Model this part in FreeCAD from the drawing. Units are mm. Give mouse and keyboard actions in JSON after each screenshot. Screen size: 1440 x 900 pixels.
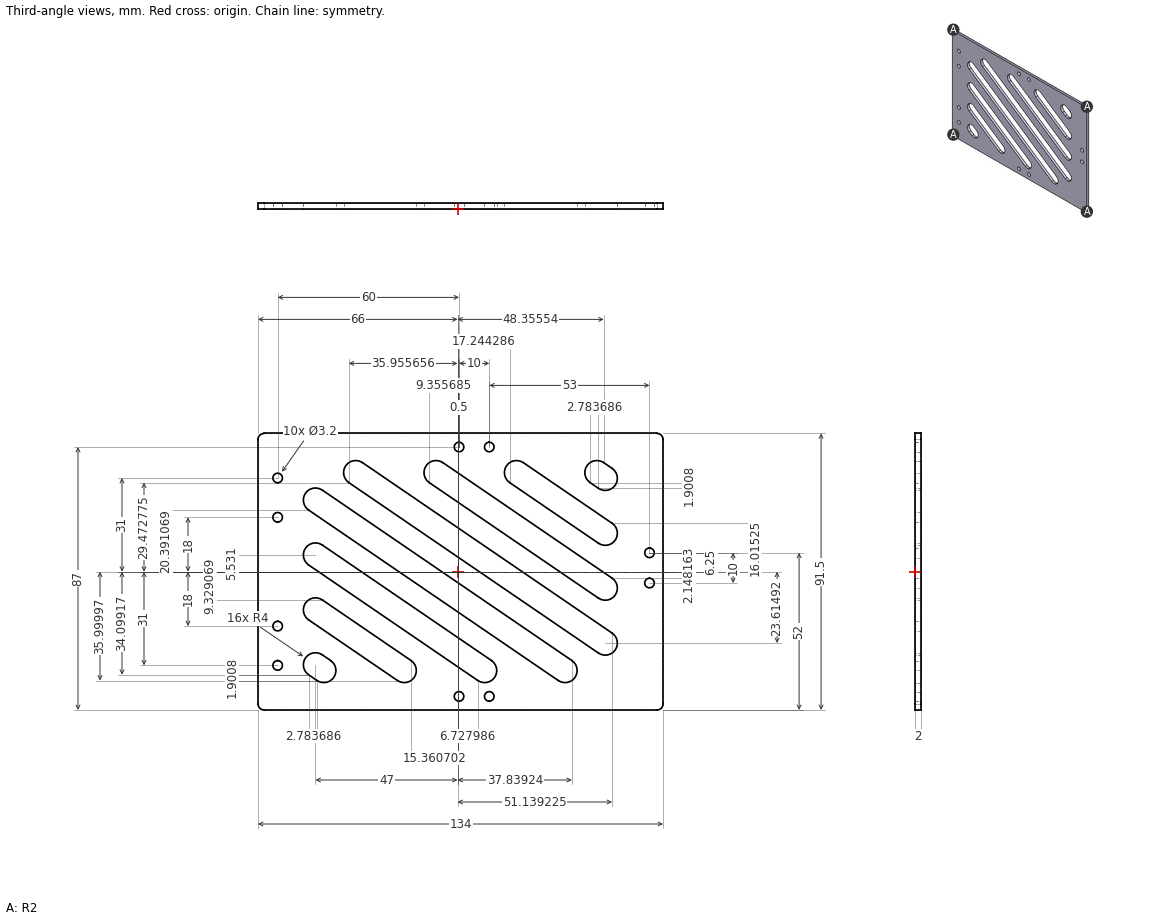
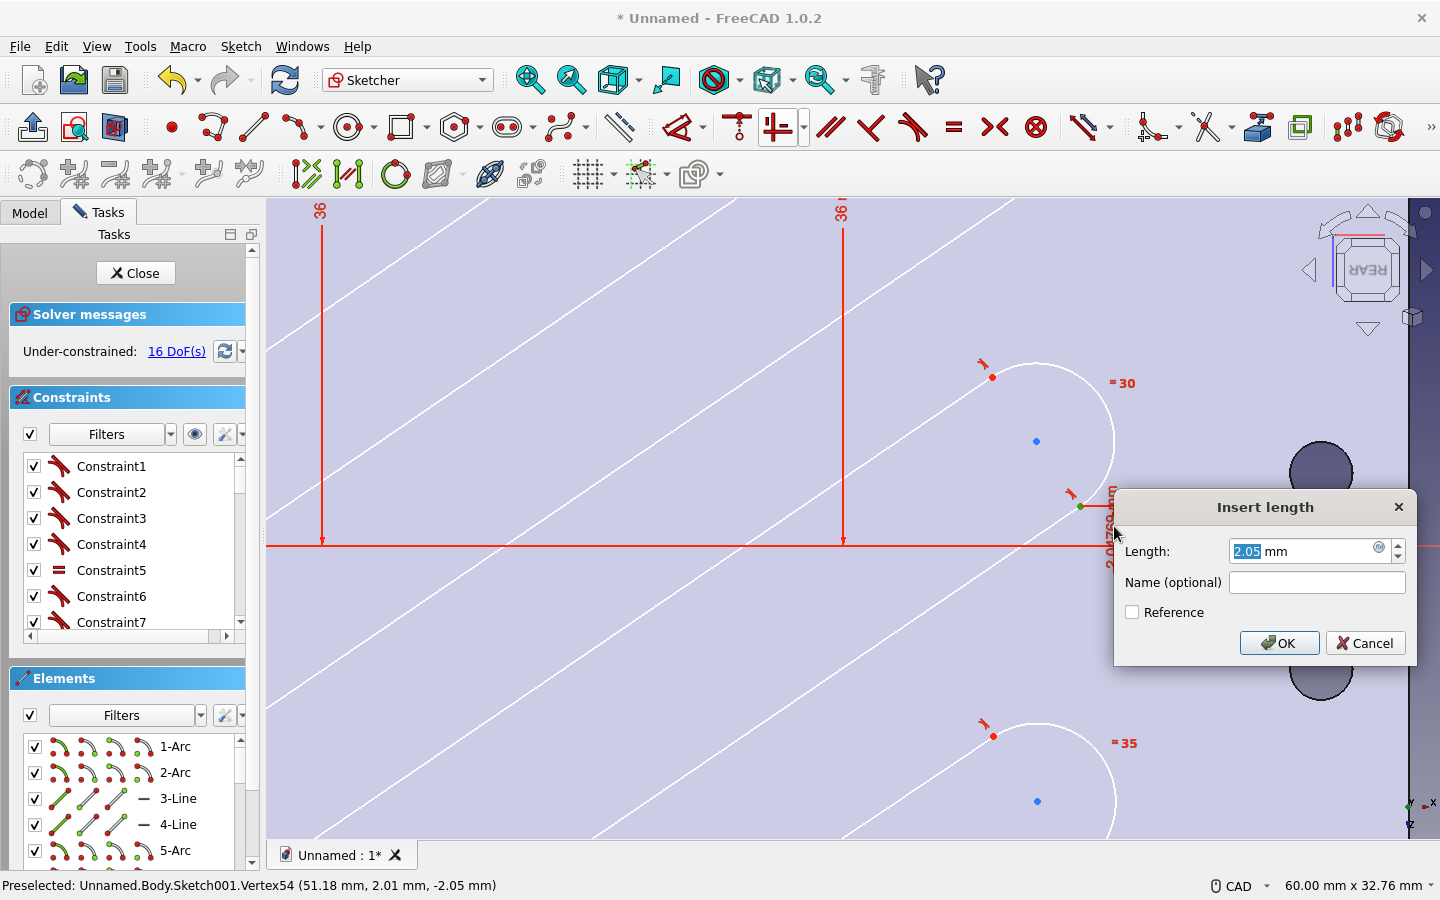
{"action": "type", "text": "2.148163"}
{"action": "key", "text": "Return"}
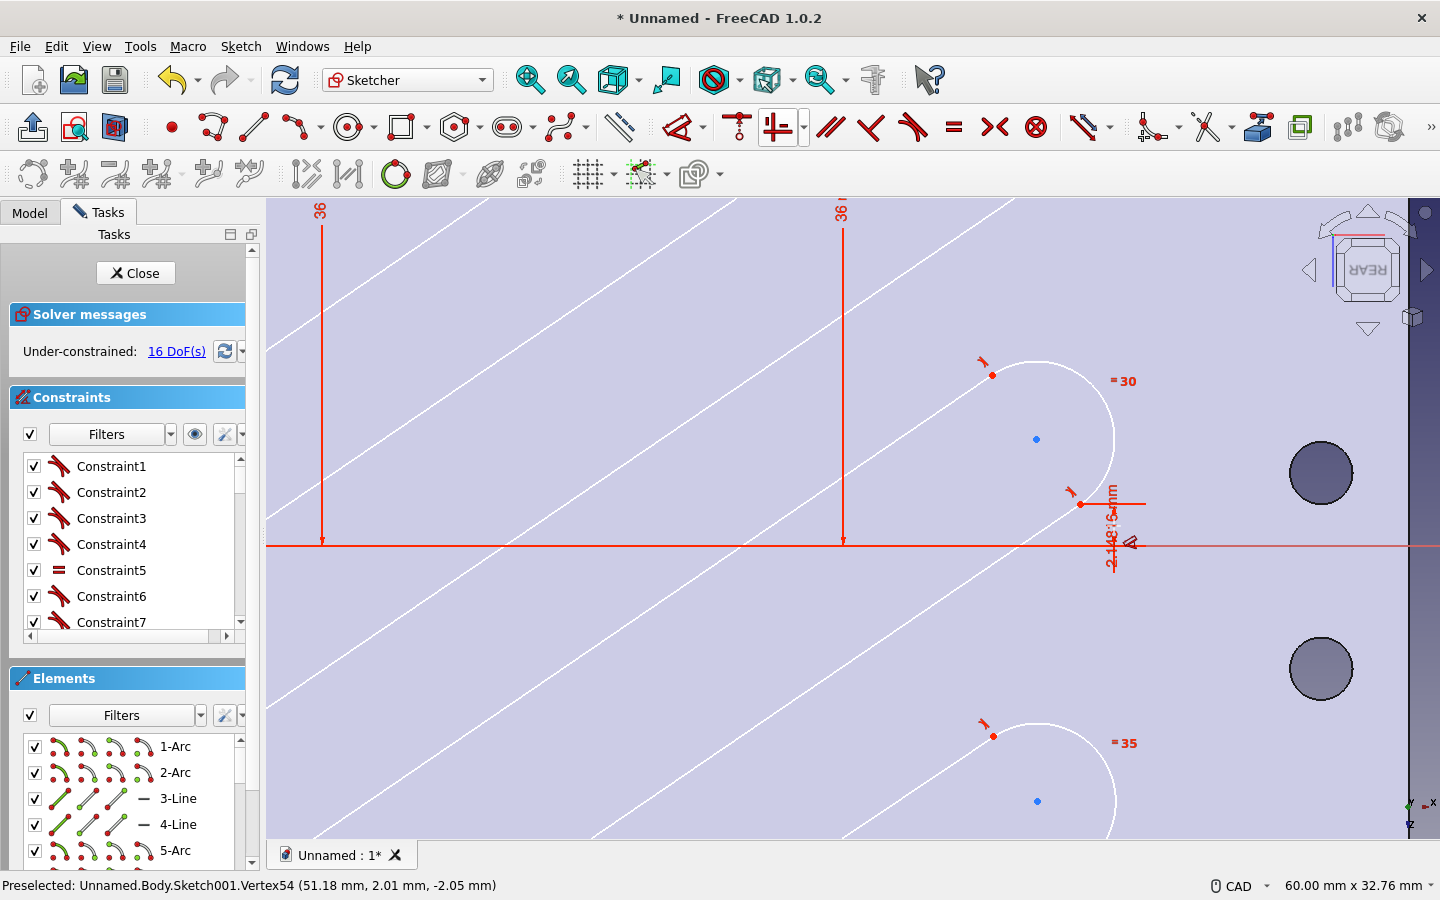
{"action": "scroll", "coordinate": [1081, 506], "scroll_direction": "down", "scroll_amount": 6}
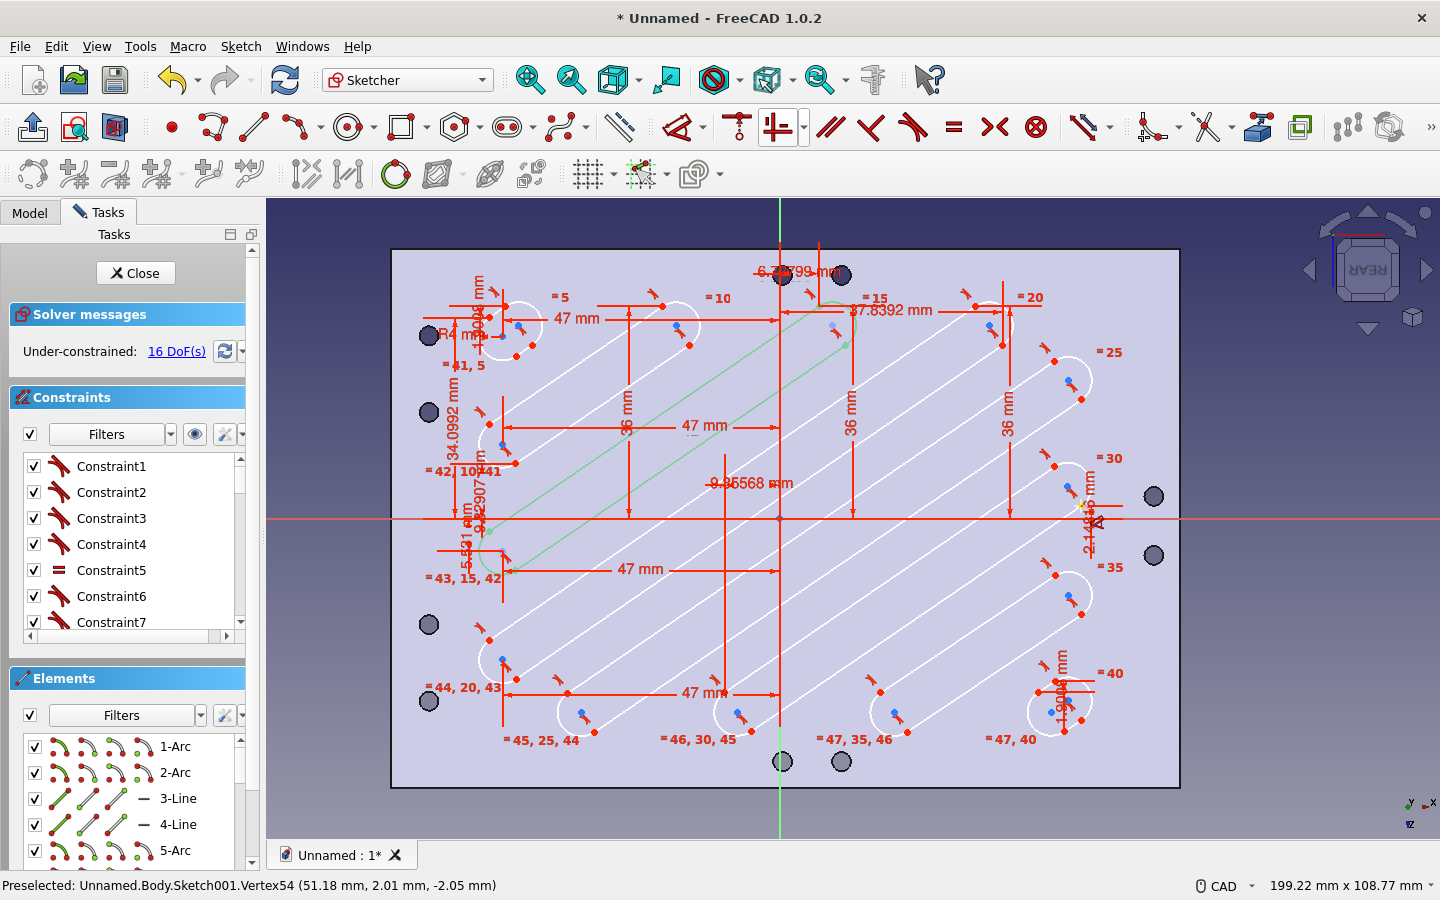
{"action": "left_click", "coordinate": [1082, 615]}
{"action": "left_click", "coordinate": [1116, 567]}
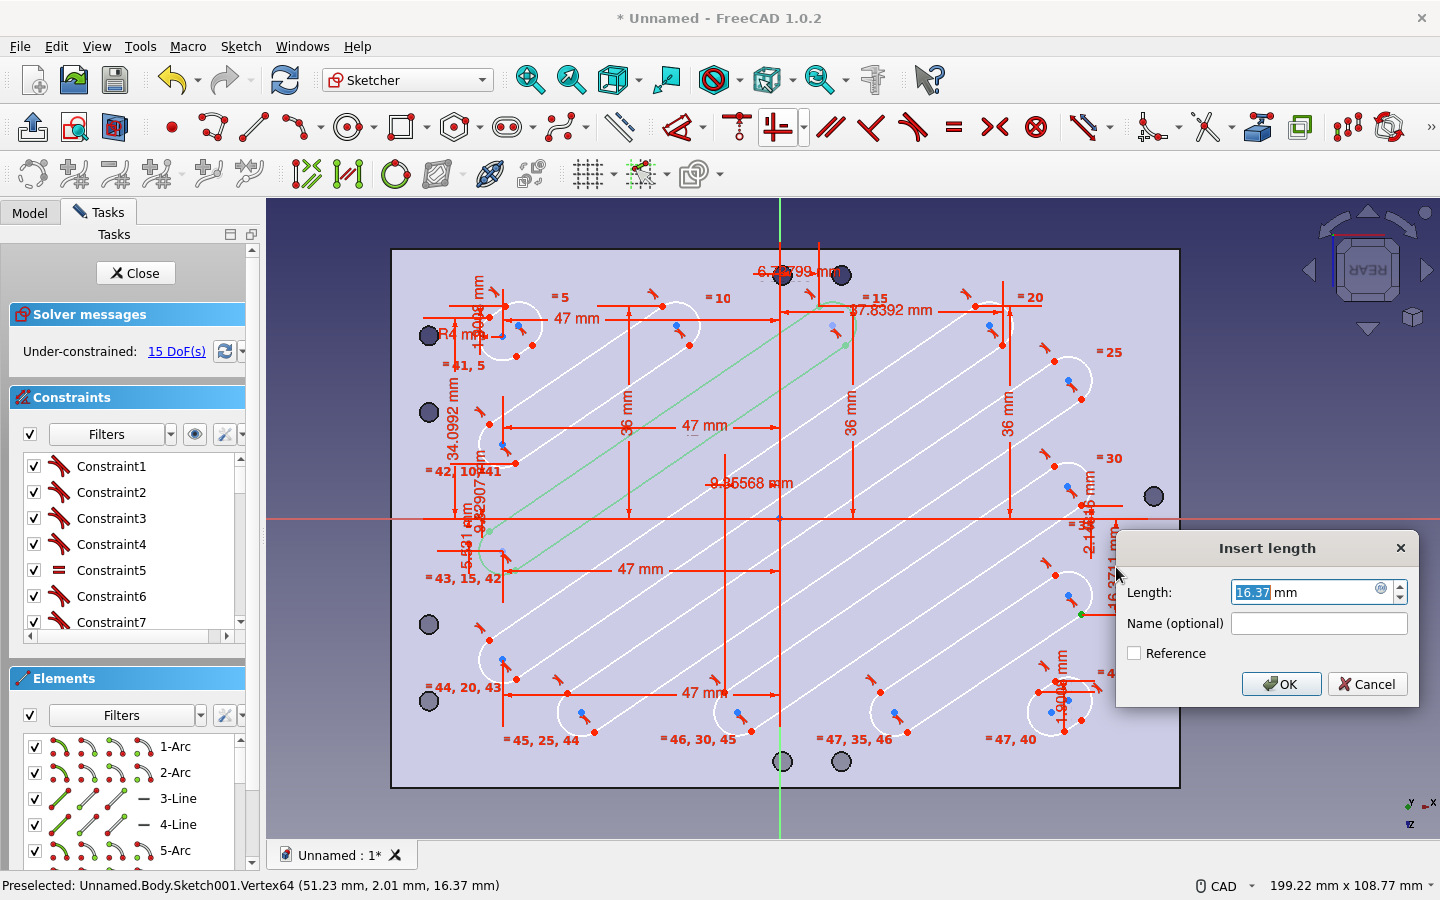
{"action": "type", "text": "16.01525"}
{"action": "key", "text": "Return"}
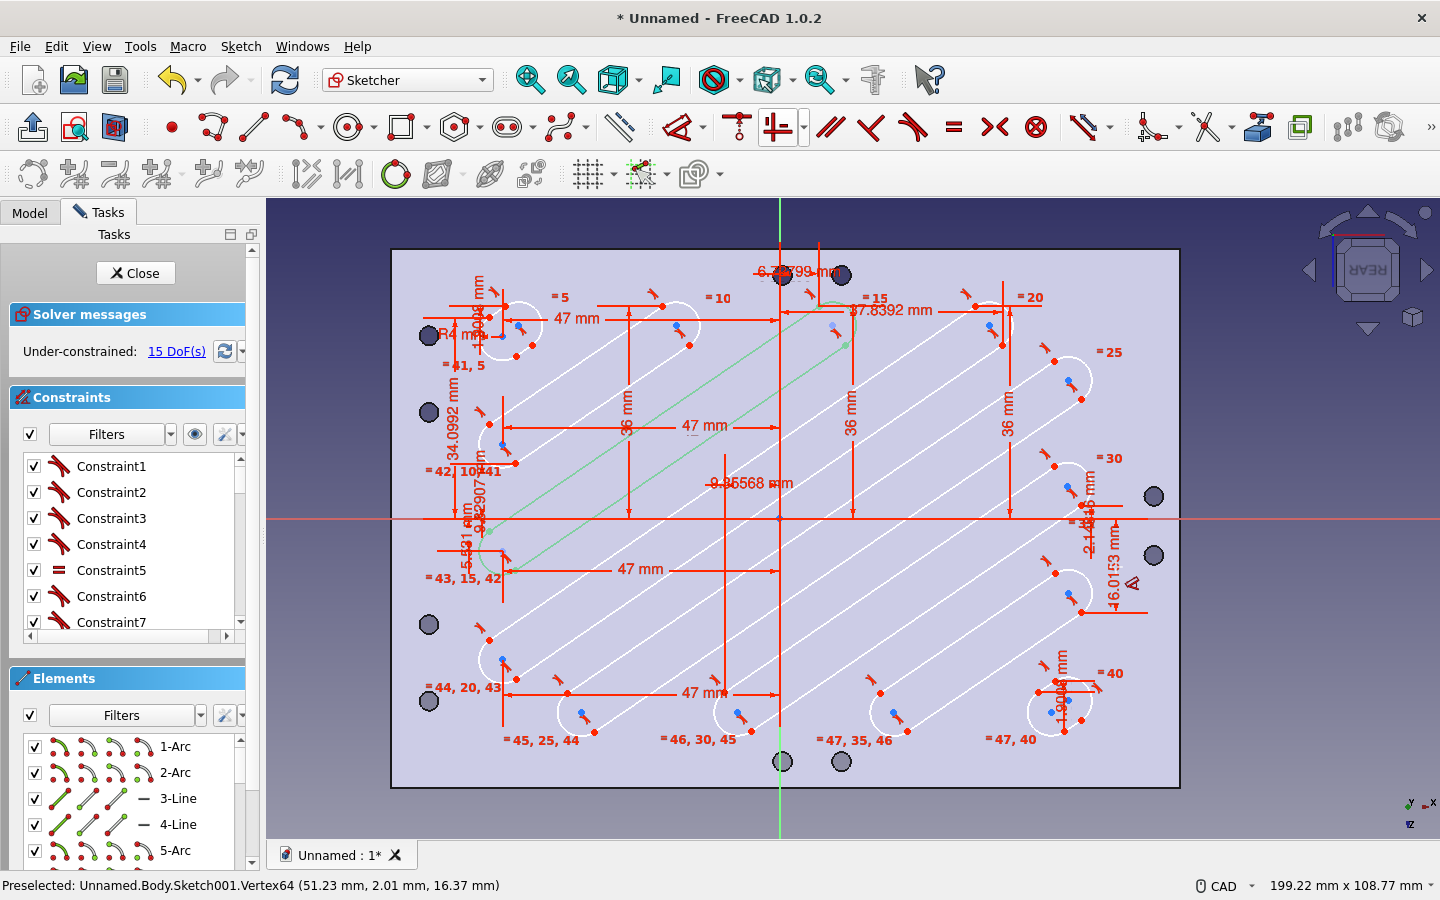
{"action": "left_click", "coordinate": [1064, 732]}
{"action": "left_click", "coordinate": [922, 766]}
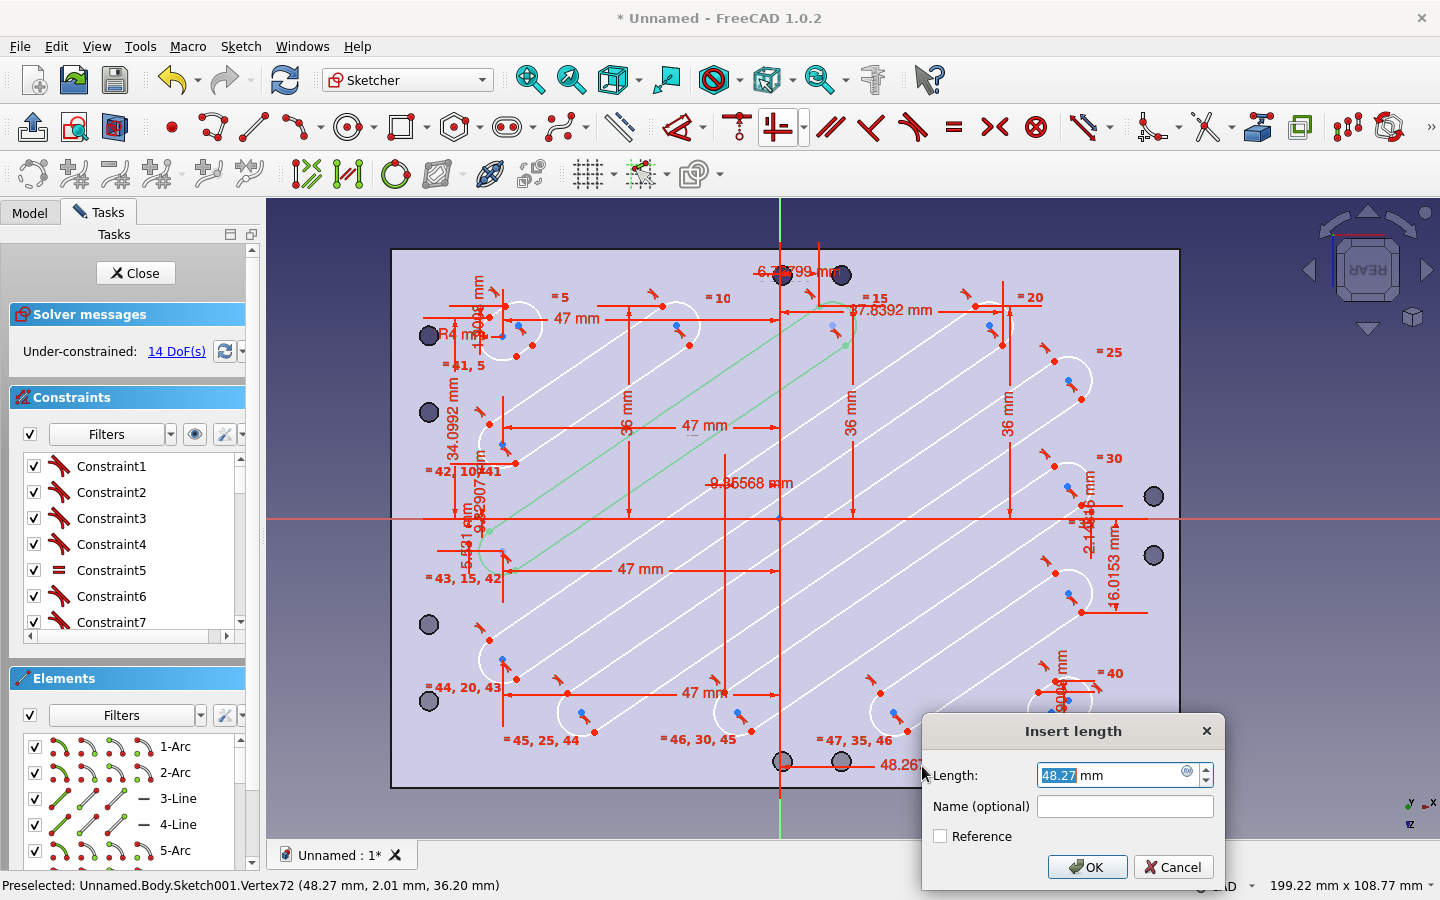
{"action": "type", "text": "48.35554"}
{"action": "key", "text": "Return"}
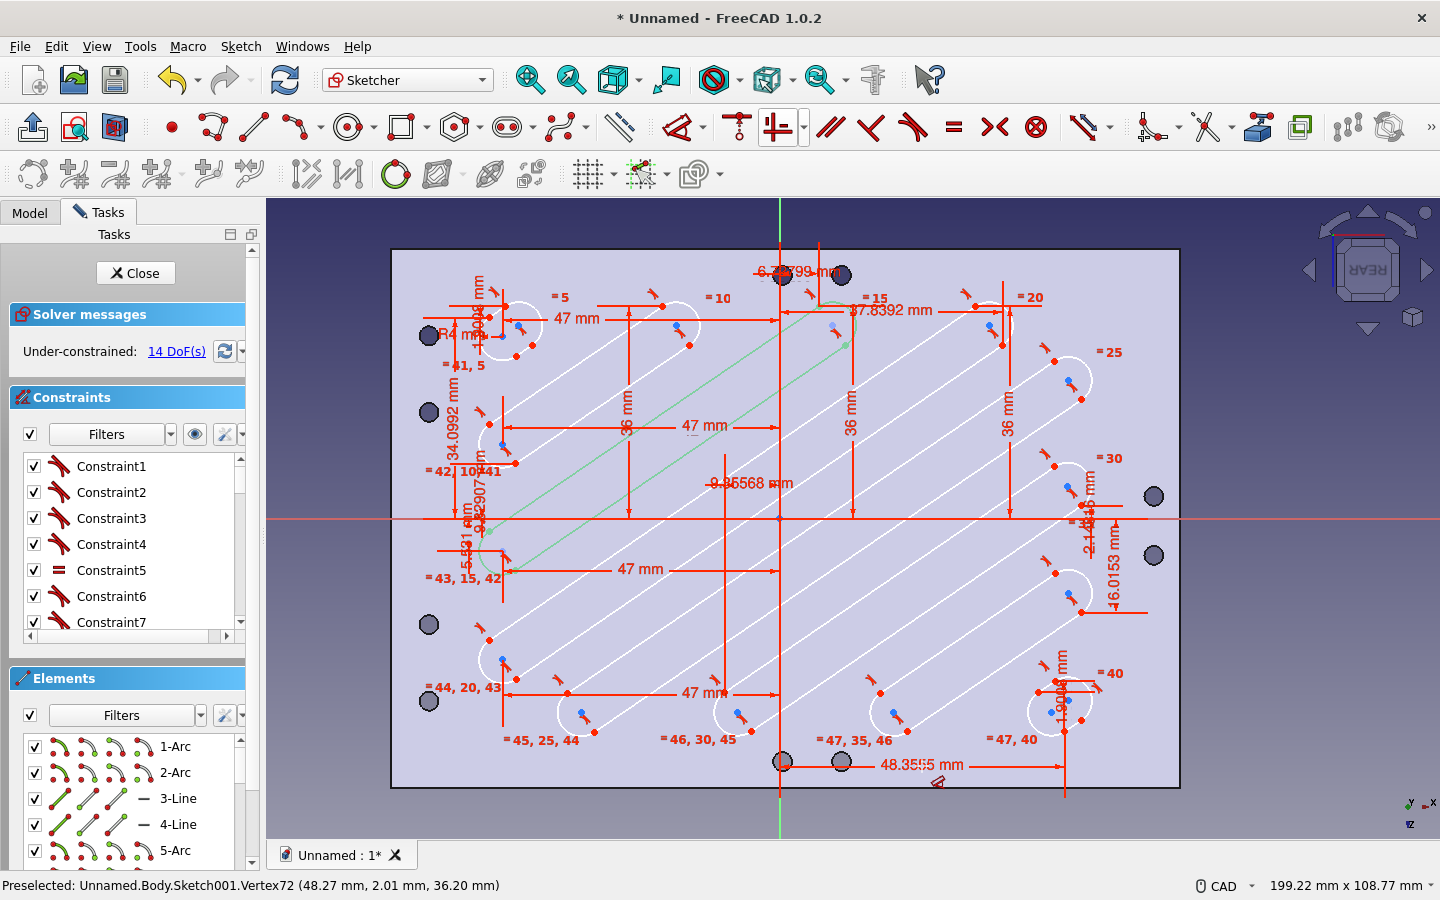
{"action": "scroll", "coordinate": [497, 312], "scroll_direction": "up", "scroll_amount": 5}